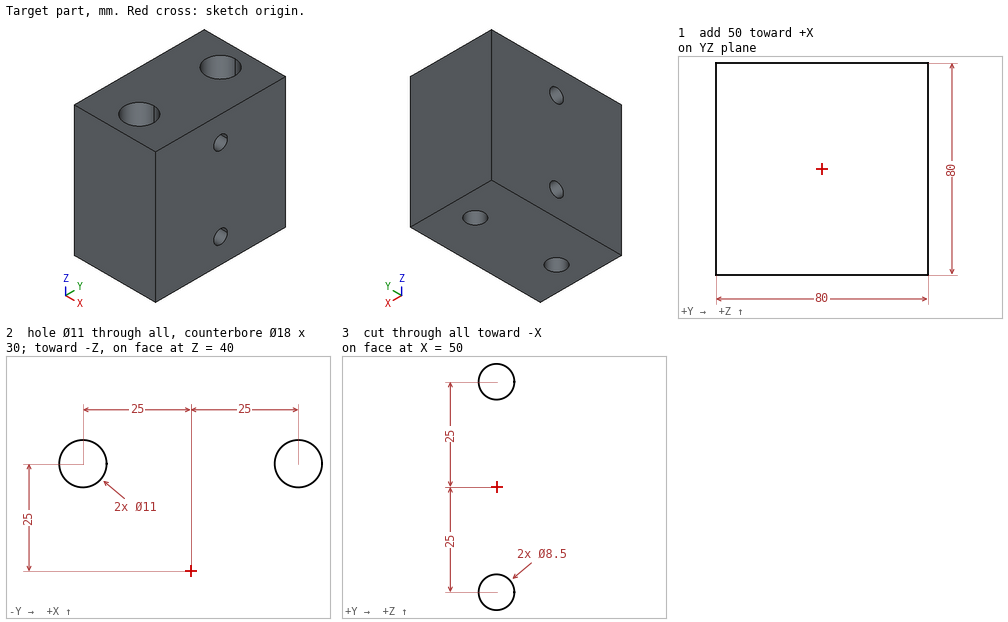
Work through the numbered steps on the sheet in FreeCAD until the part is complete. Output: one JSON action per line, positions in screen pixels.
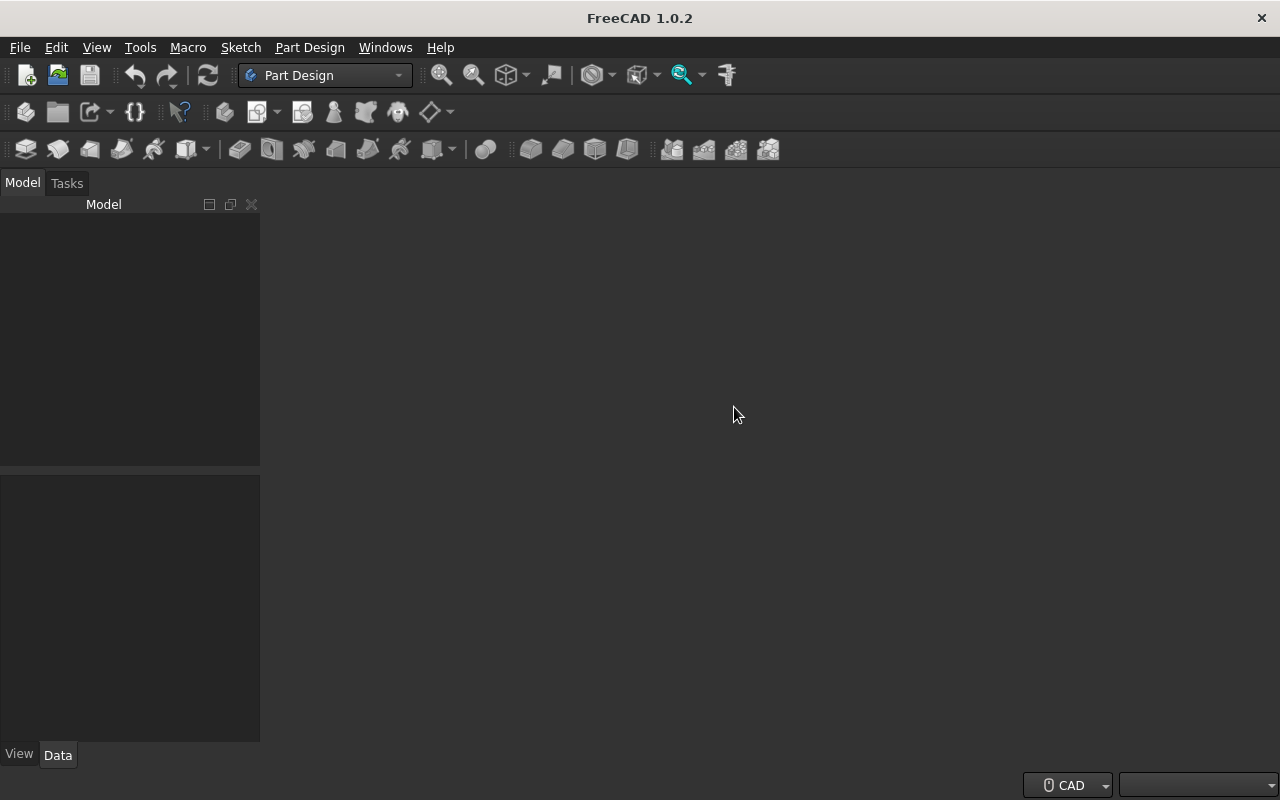
{"action": "left_click", "coordinate": [26, 76]}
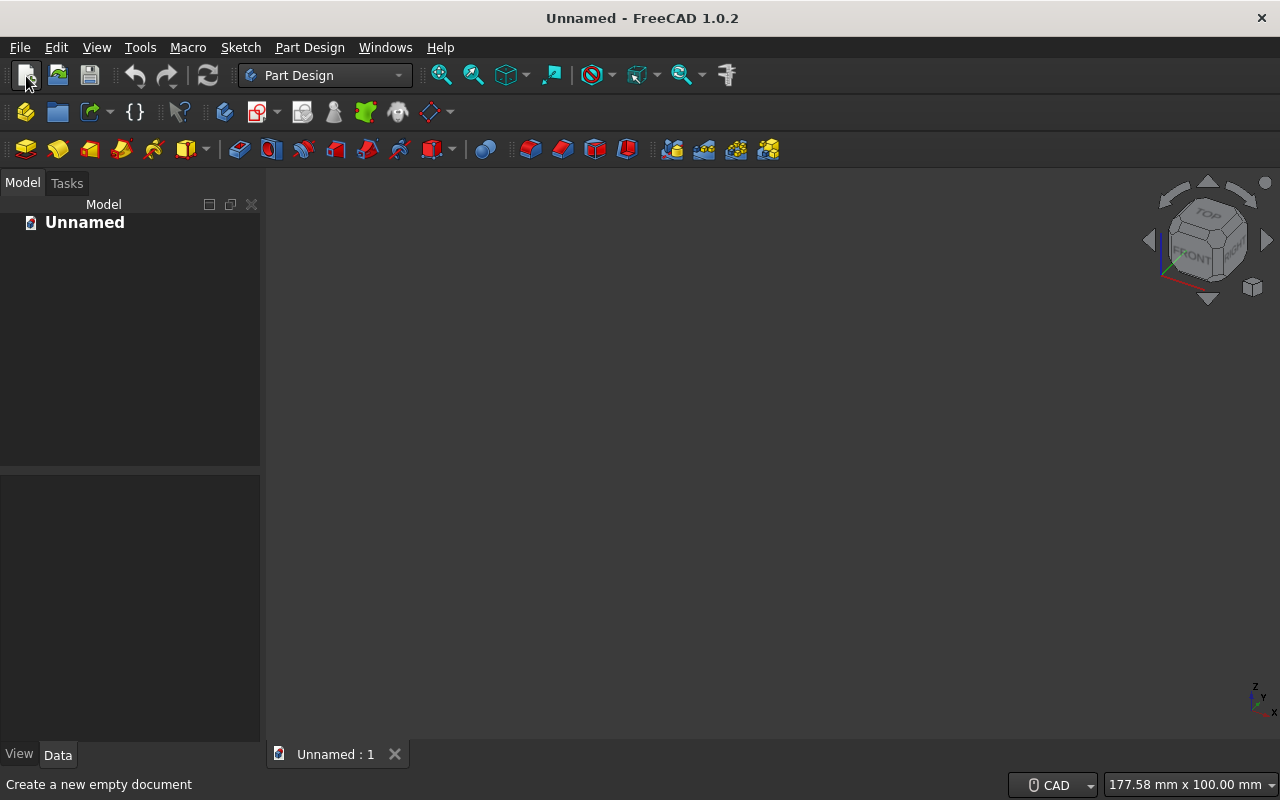
{"action": "left_click", "coordinate": [258, 112]}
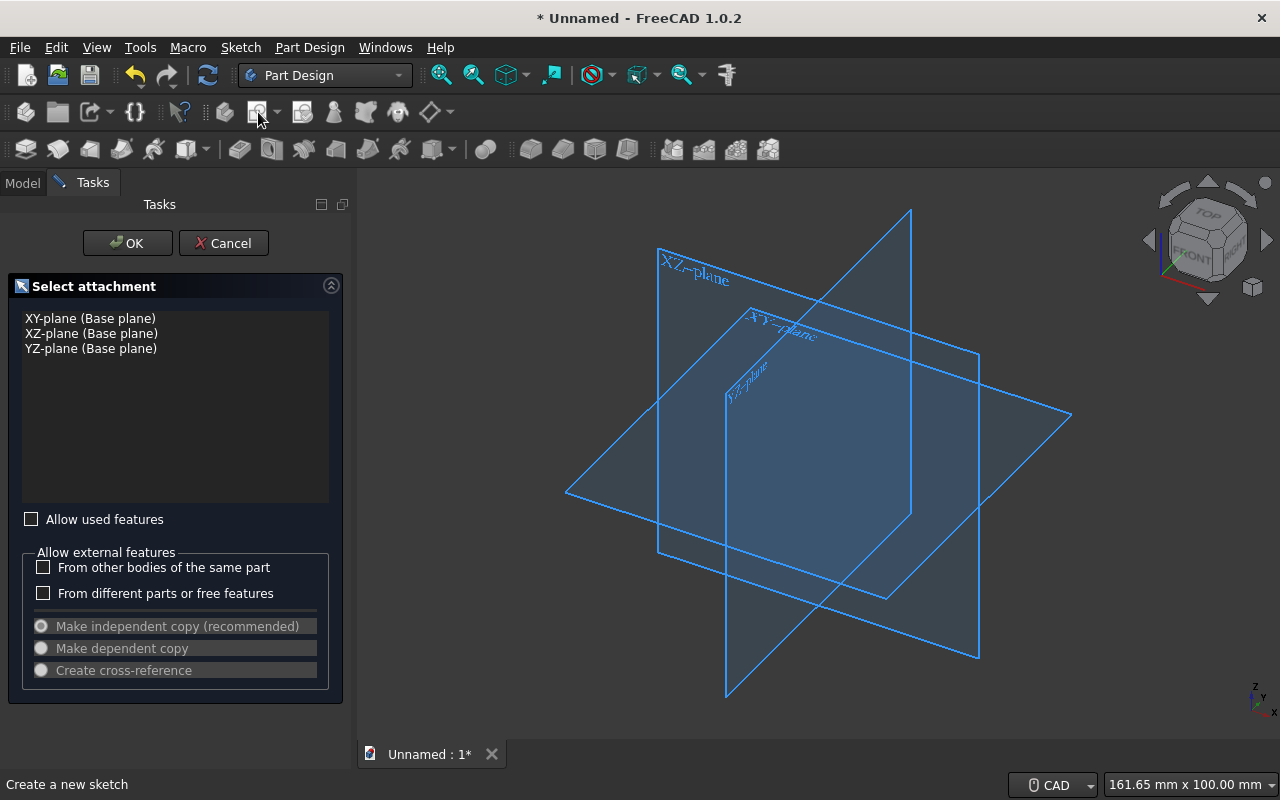
{"action": "left_click", "coordinate": [82, 348]}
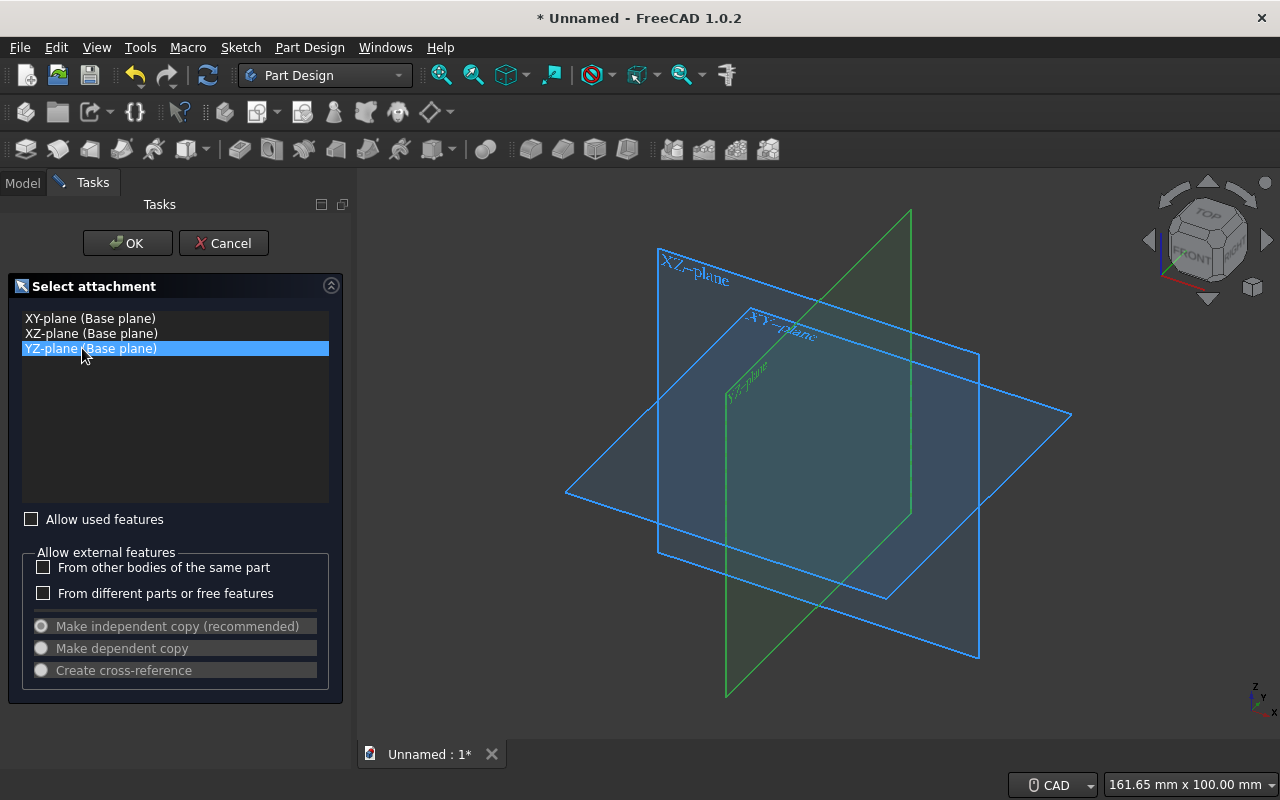
{"action": "left_click", "coordinate": [128, 243]}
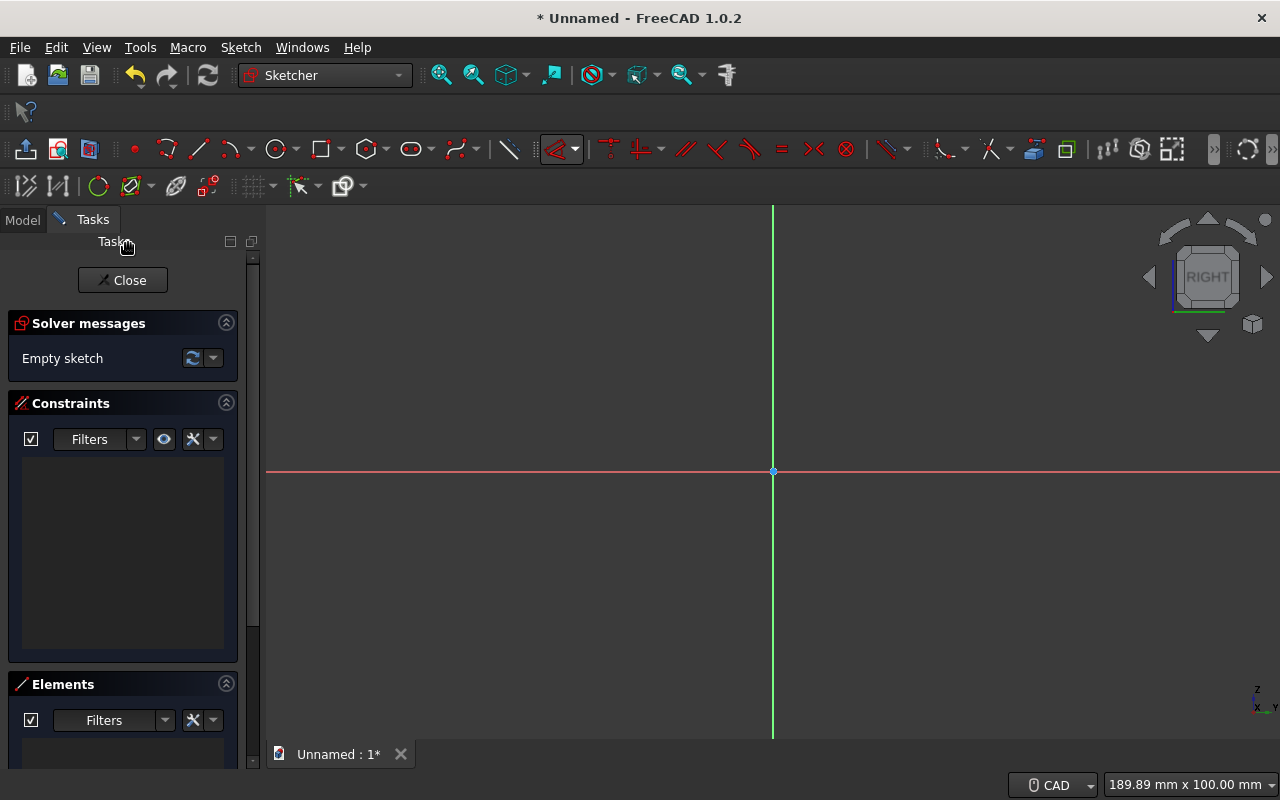
{"action": "key", "text": "g v"}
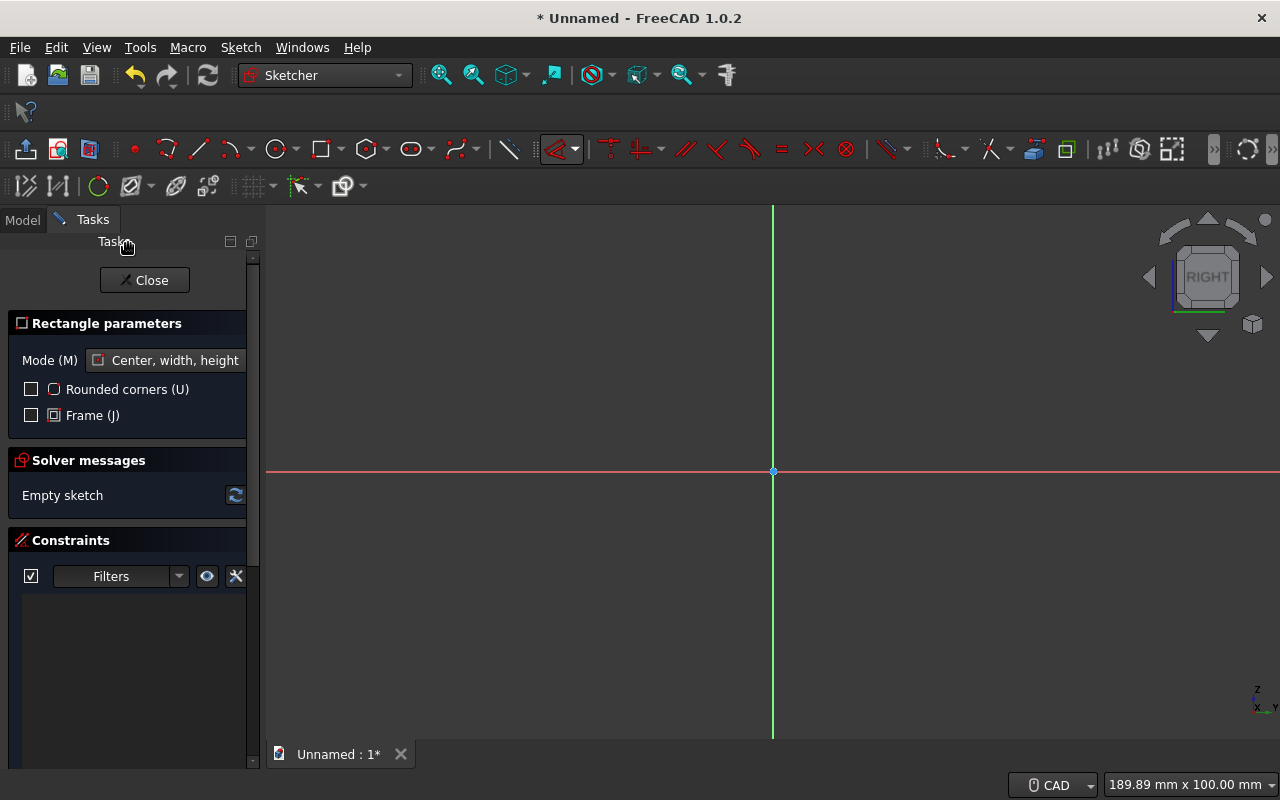
{"action": "left_click", "coordinate": [773, 472]}
{"action": "left_click", "coordinate": [987, 258]}
{"action": "key", "text": "Escape"}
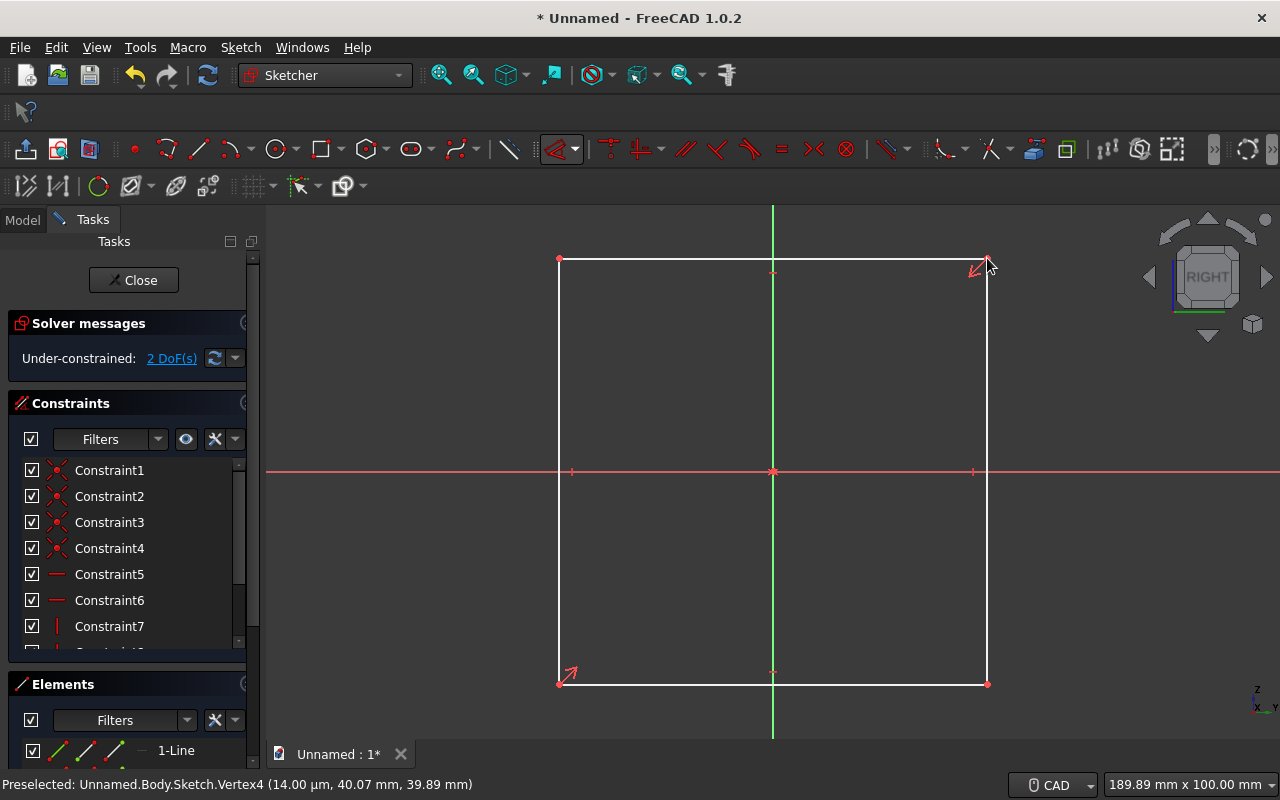
{"action": "left_click", "coordinate": [556, 150]}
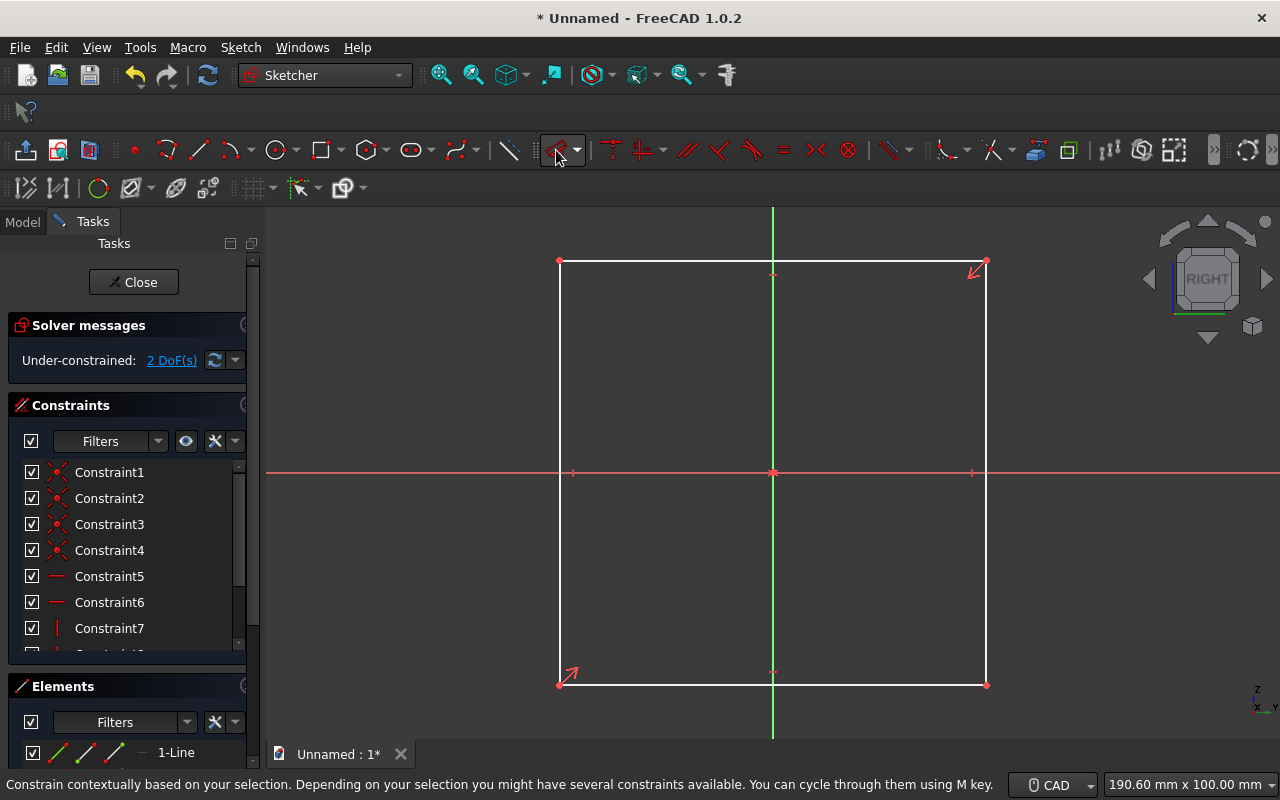
{"action": "left_click", "coordinate": [688, 685]}
{"action": "left_click", "coordinate": [675, 651]}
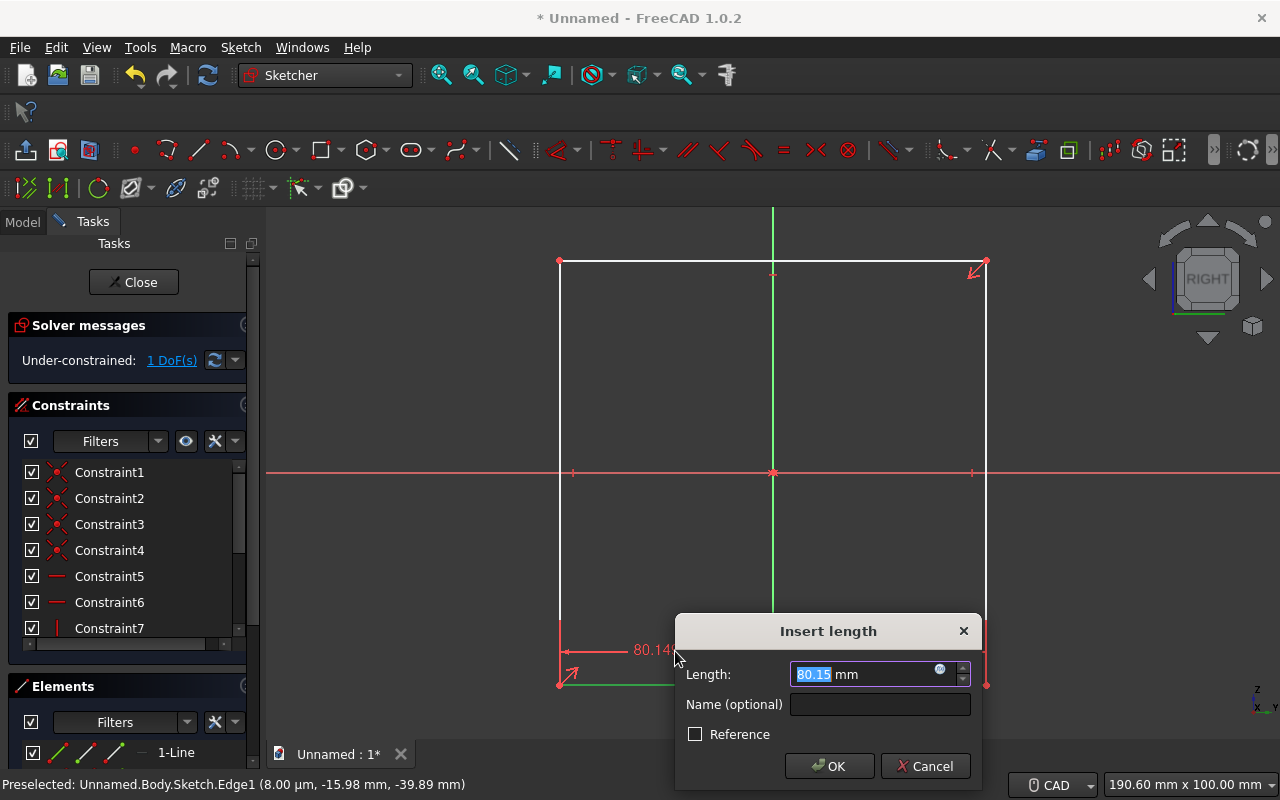
{"action": "type", "text": "80"}
{"action": "key", "text": "Return"}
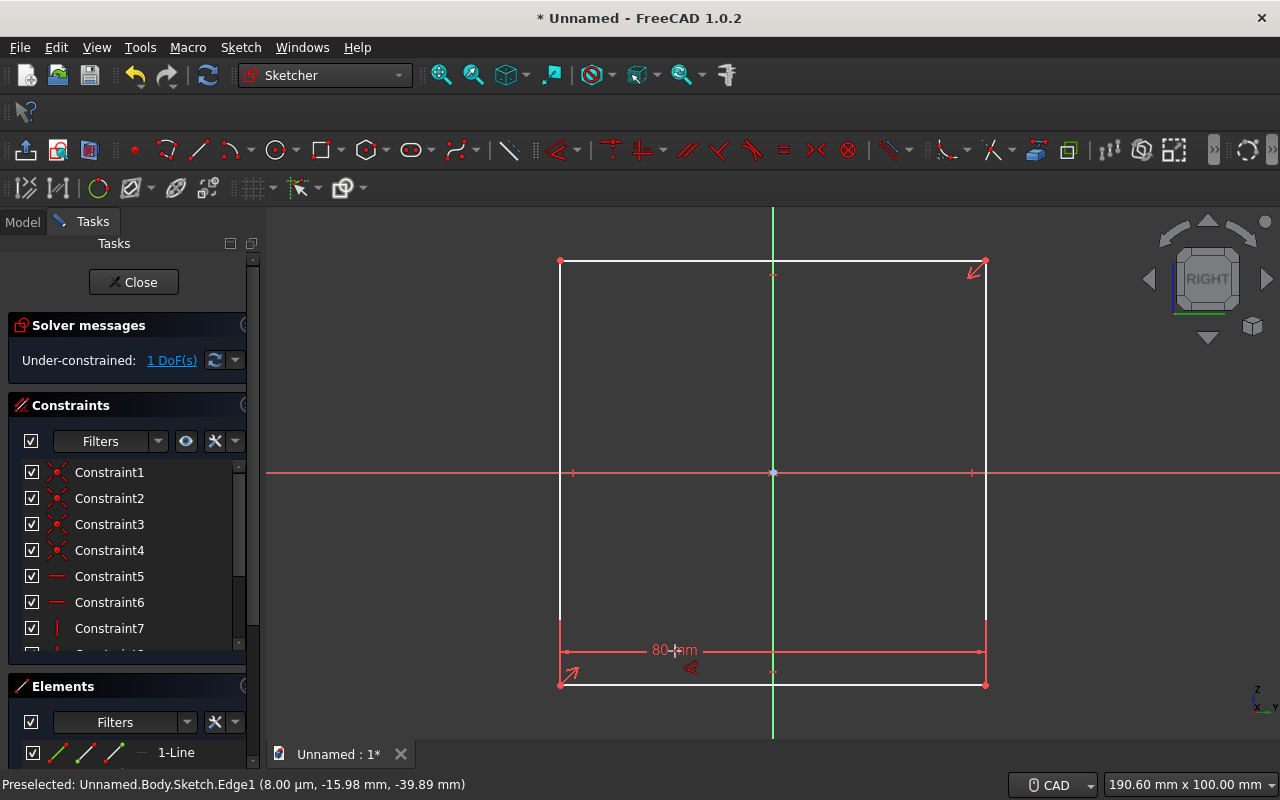
{"action": "left_click", "coordinate": [986, 558]}
{"action": "left_click", "coordinate": [1020, 375]}